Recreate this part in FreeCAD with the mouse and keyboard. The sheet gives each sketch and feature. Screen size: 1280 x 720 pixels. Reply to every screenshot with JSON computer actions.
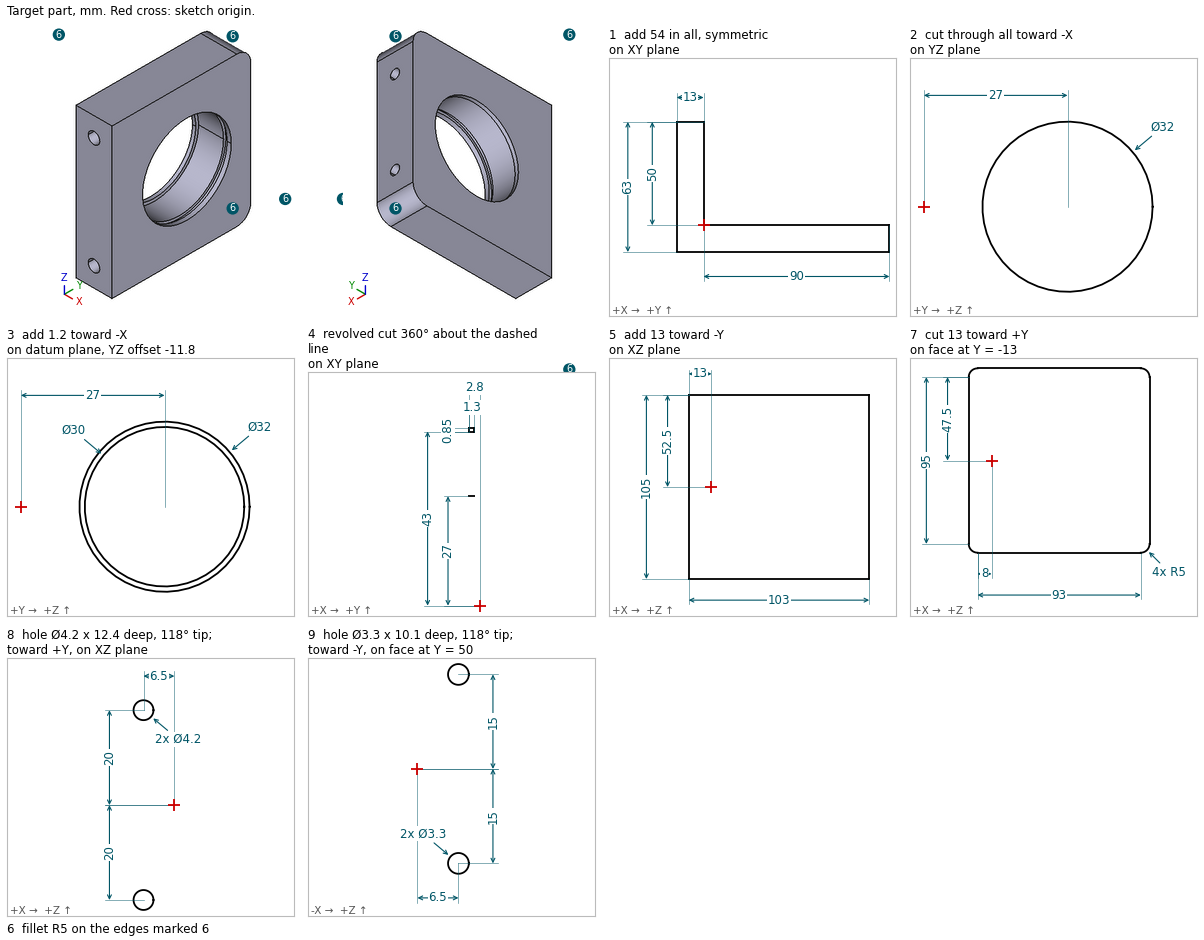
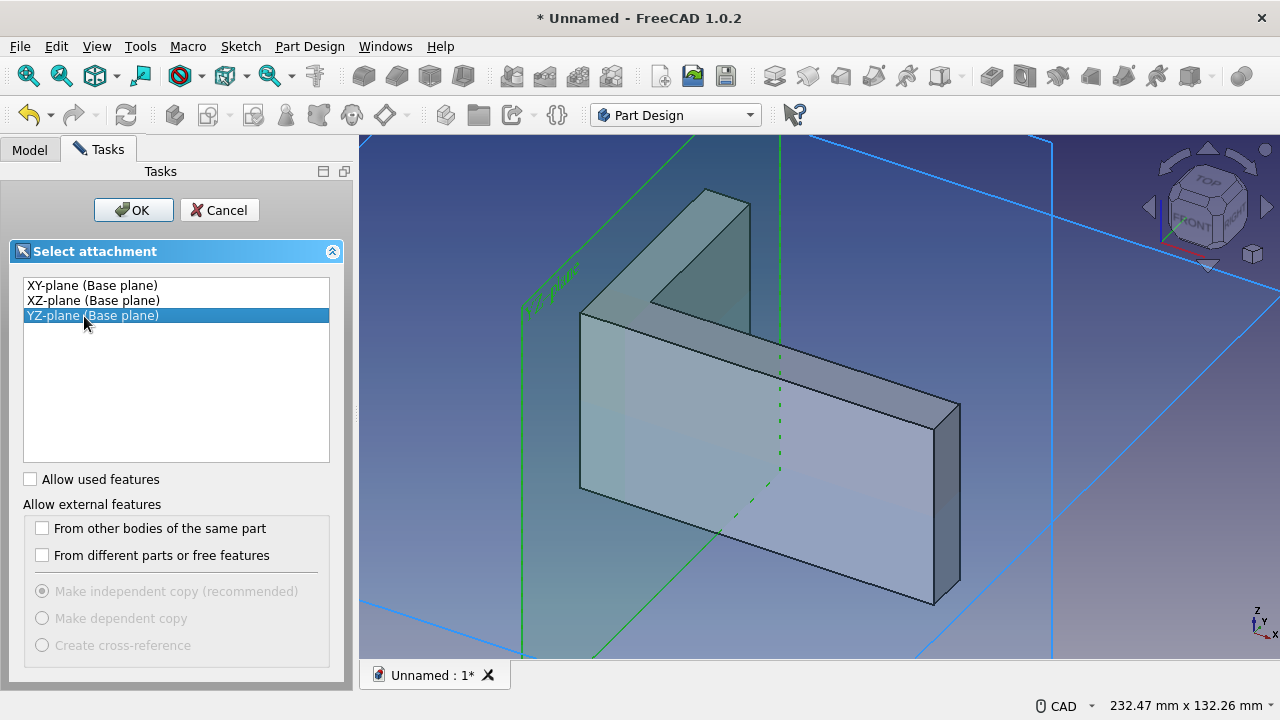
{"action": "left_click", "coordinate": [134, 210]}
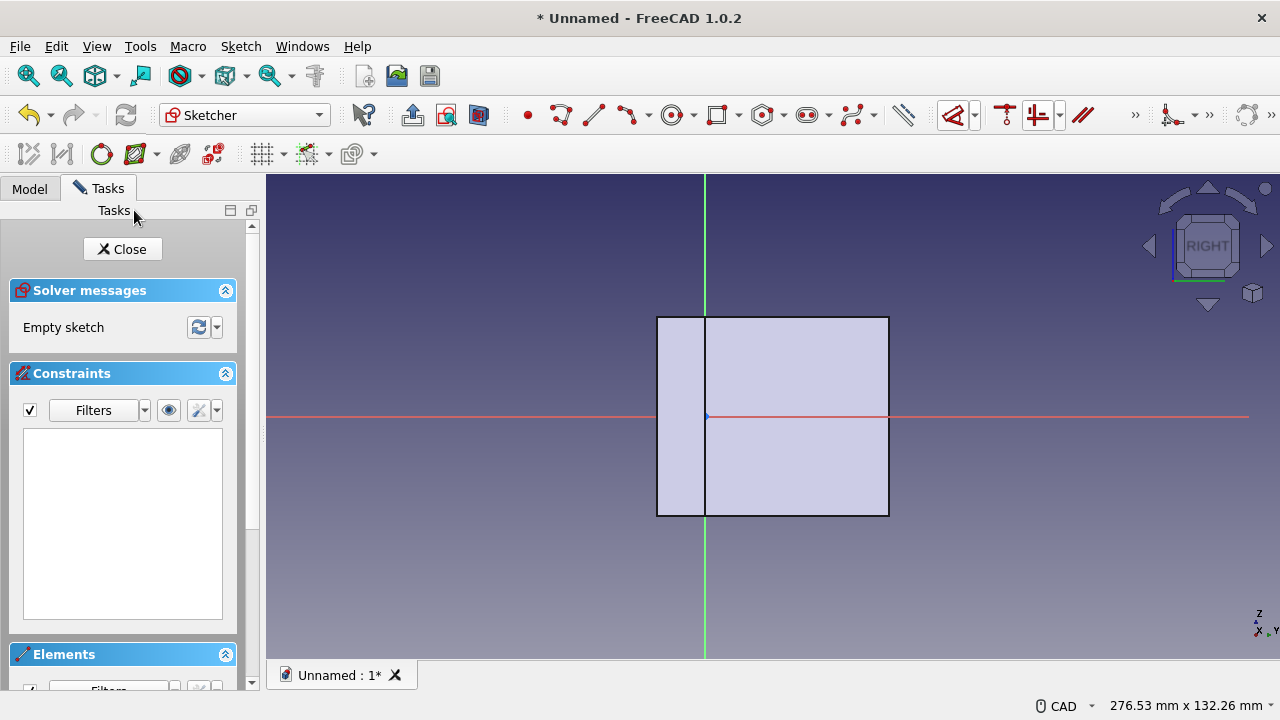
{"action": "left_click", "coordinate": [479, 116]}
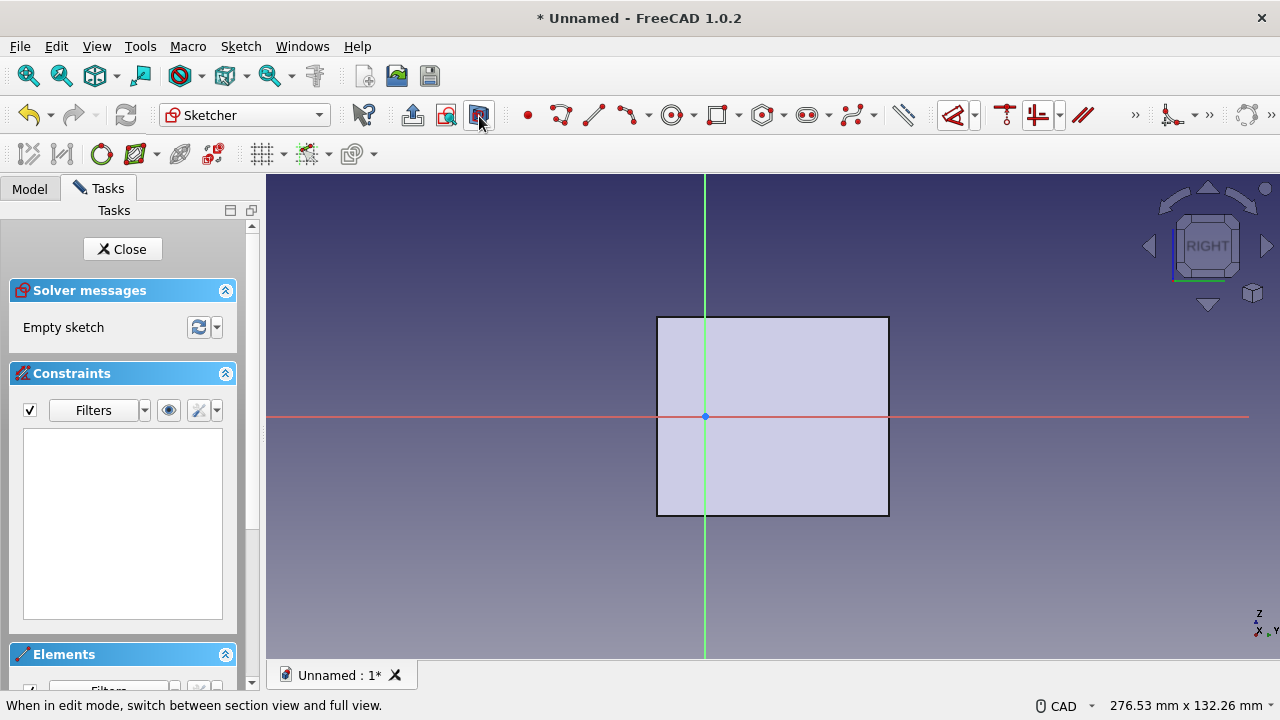
{"action": "scroll", "coordinate": [830, 416], "scroll_direction": "up", "scroll_amount": 5}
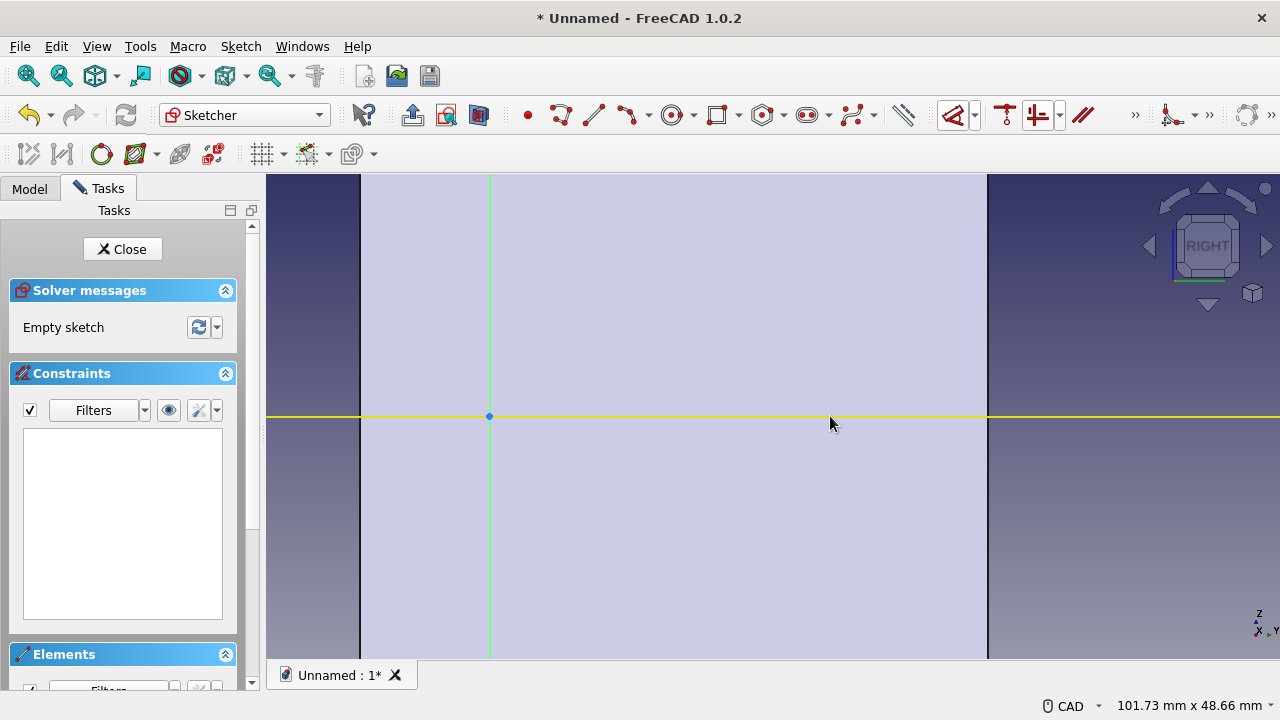
{"action": "left_click", "coordinate": [672, 116]}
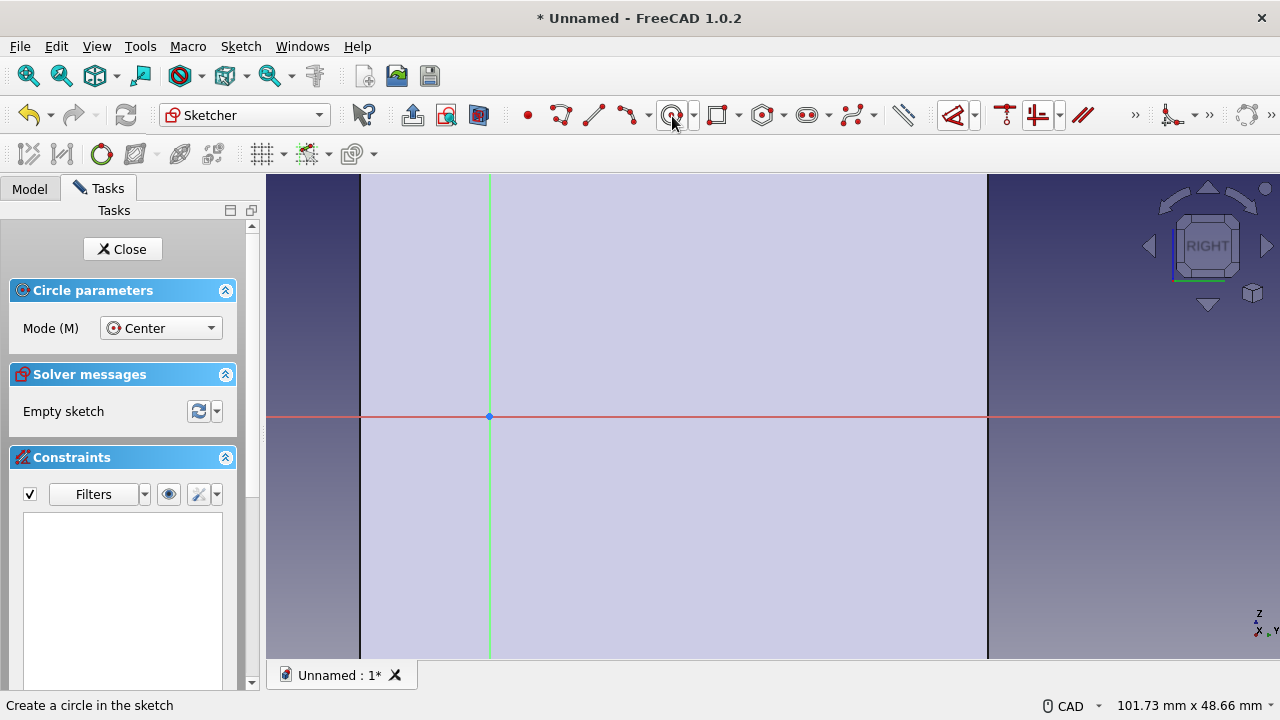
{"action": "left_click", "coordinate": [759, 416]}
{"action": "left_click", "coordinate": [872, 304]}
{"action": "key", "text": "Escape"}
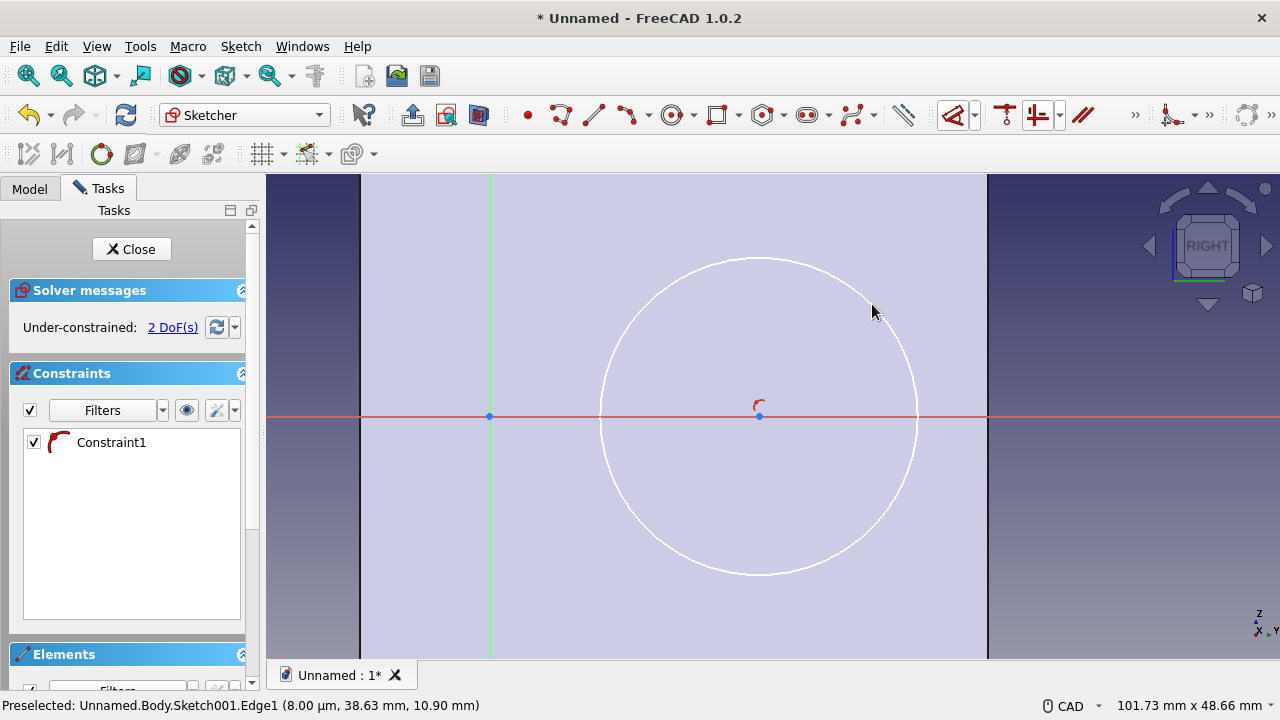
{"action": "left_click", "coordinate": [871, 304]}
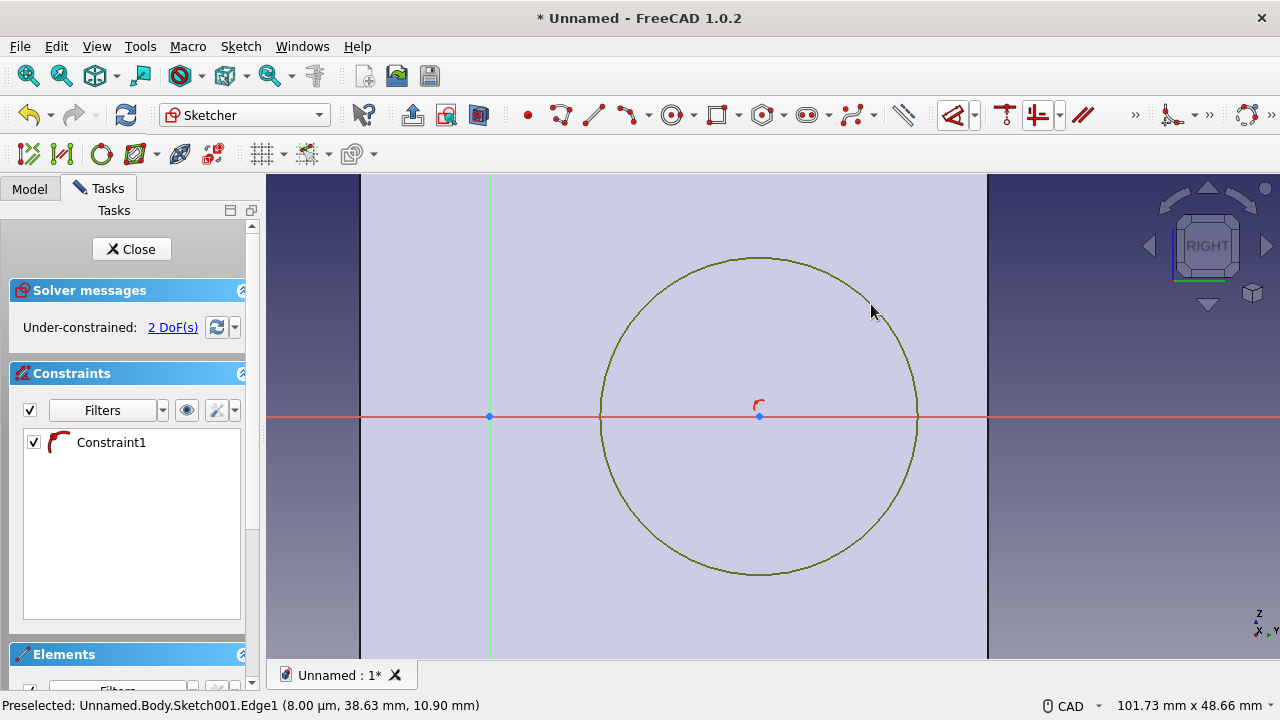
{"action": "key", "text": "k o"}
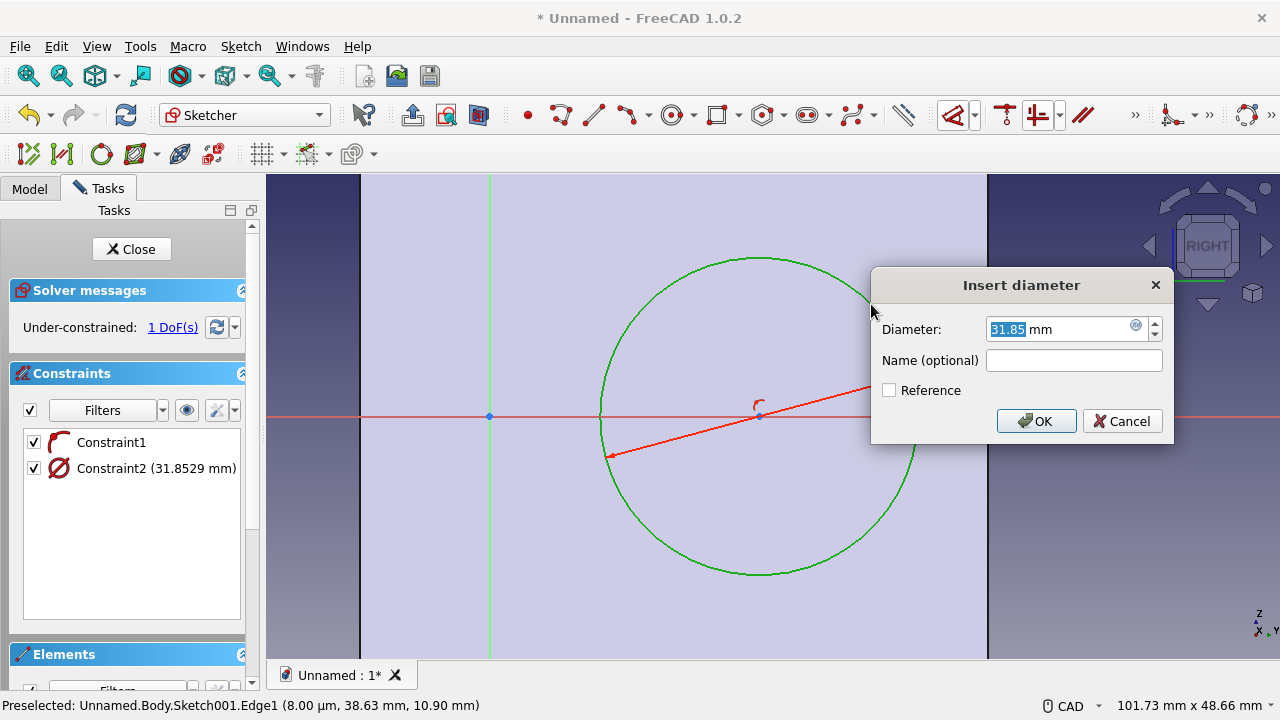
{"action": "type", "text": "32"}
{"action": "key", "text": "Return"}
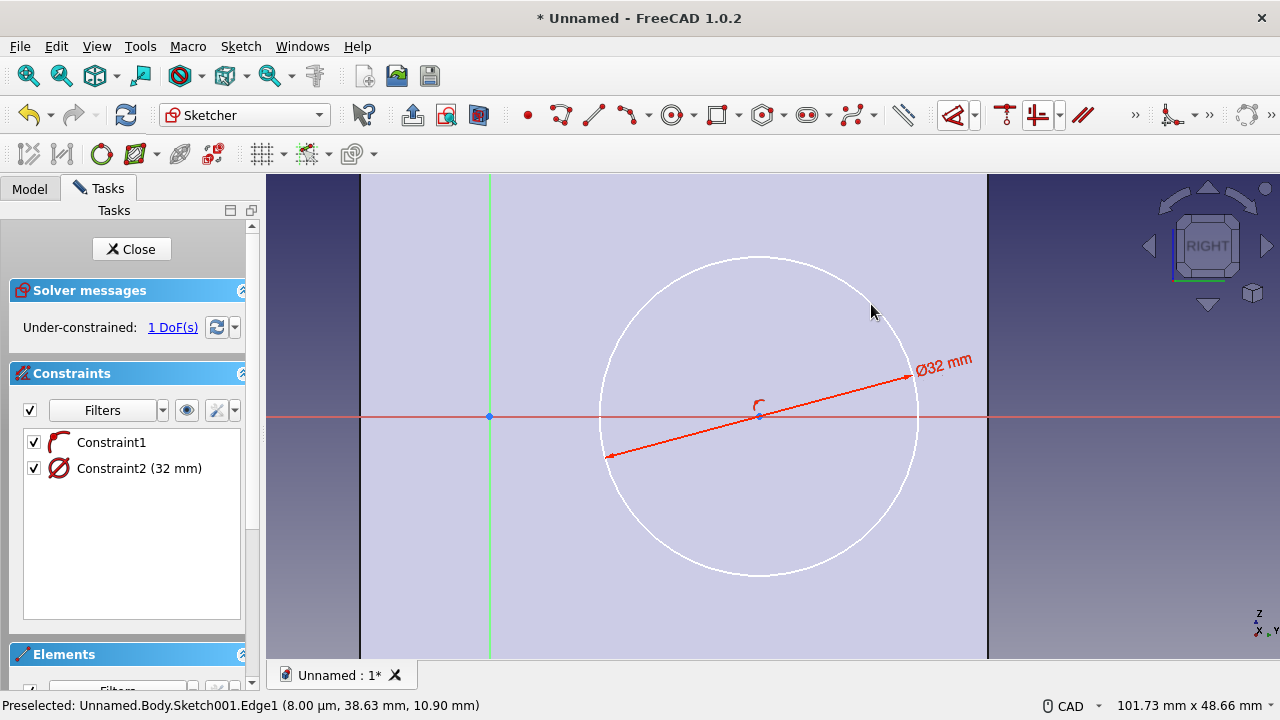
{"action": "left_click", "coordinate": [759, 416]}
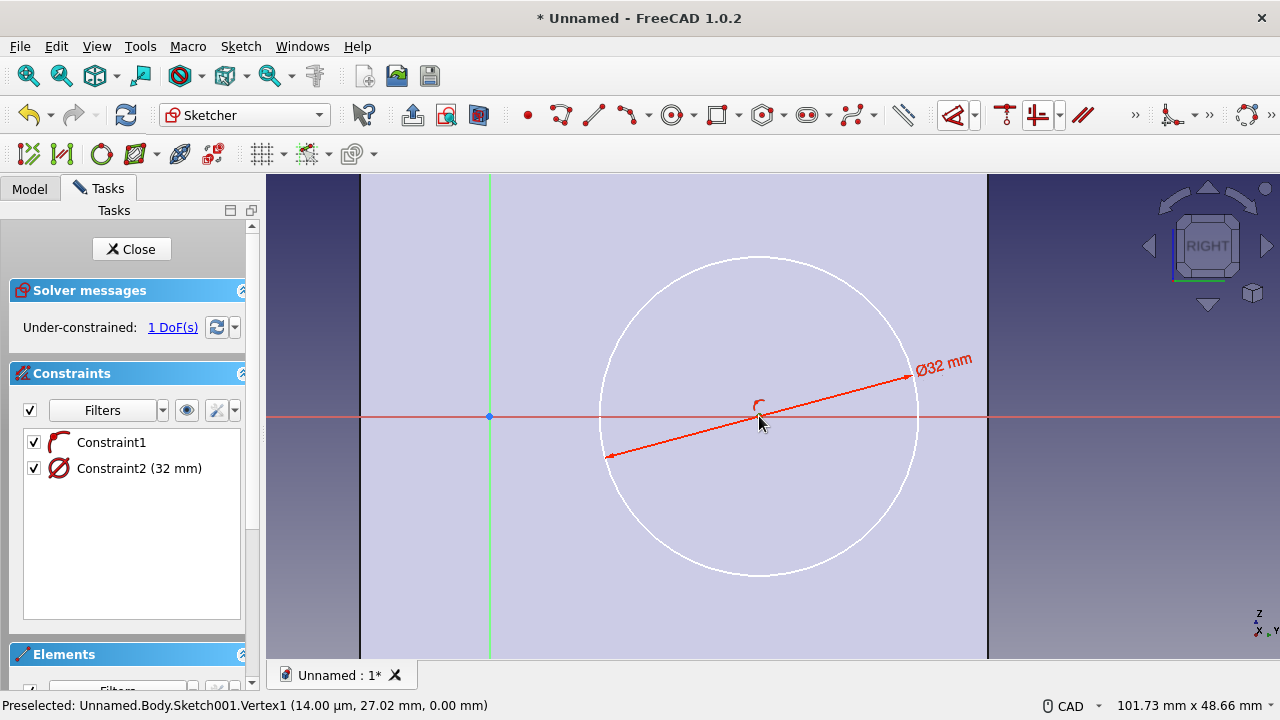
{"action": "left_click", "coordinate": [974, 116]}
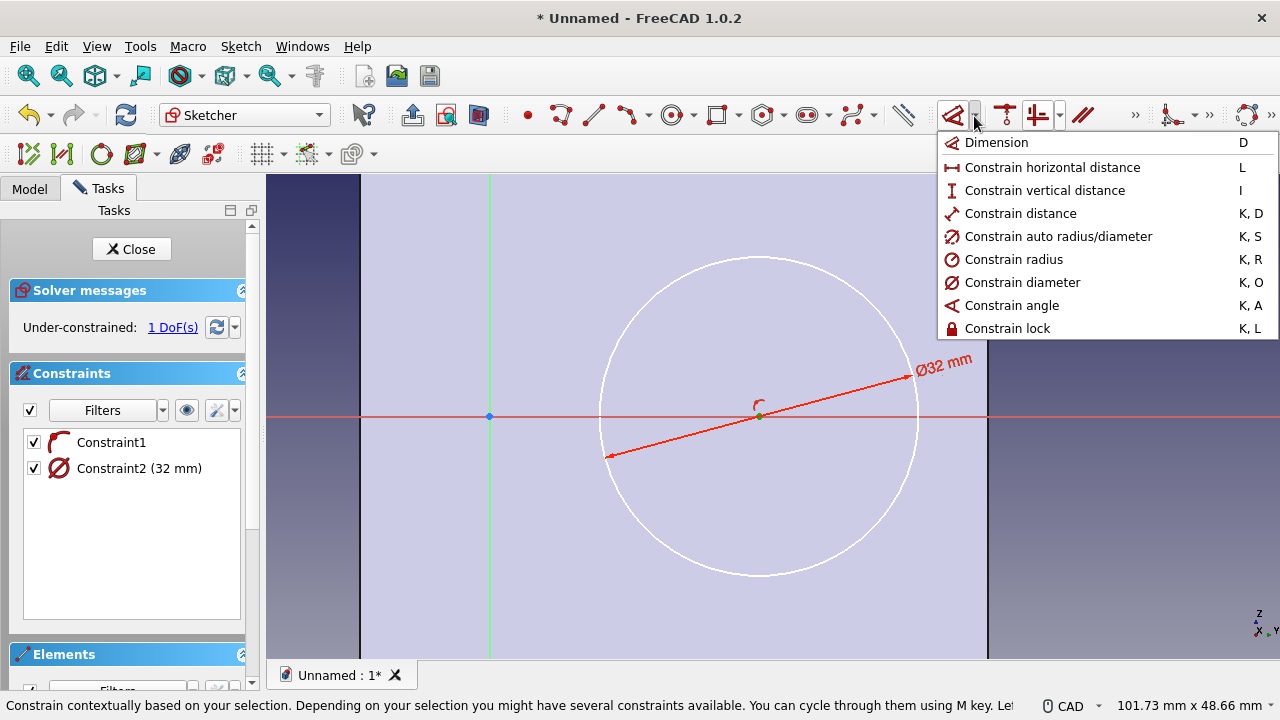
{"action": "left_click", "coordinate": [1108, 168]}